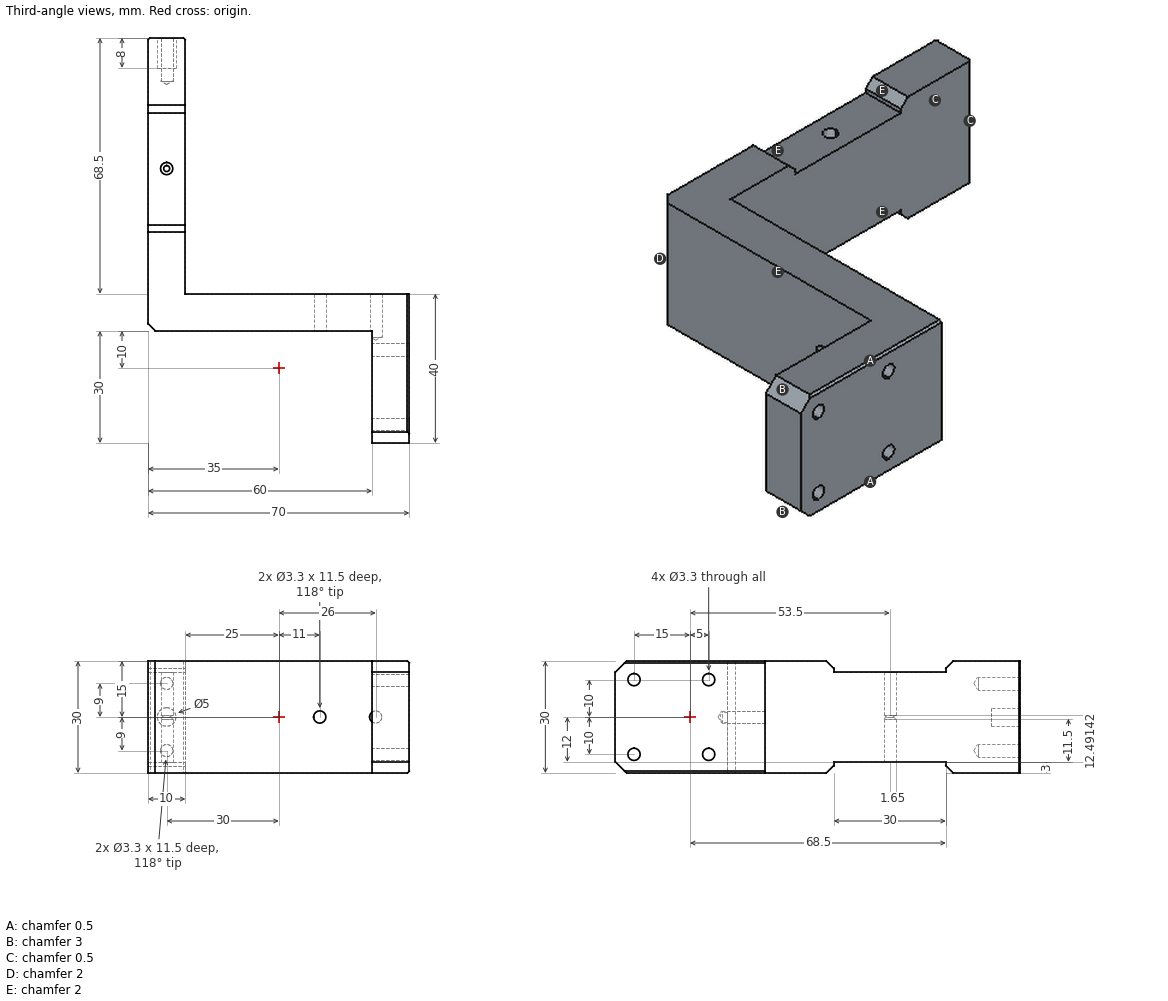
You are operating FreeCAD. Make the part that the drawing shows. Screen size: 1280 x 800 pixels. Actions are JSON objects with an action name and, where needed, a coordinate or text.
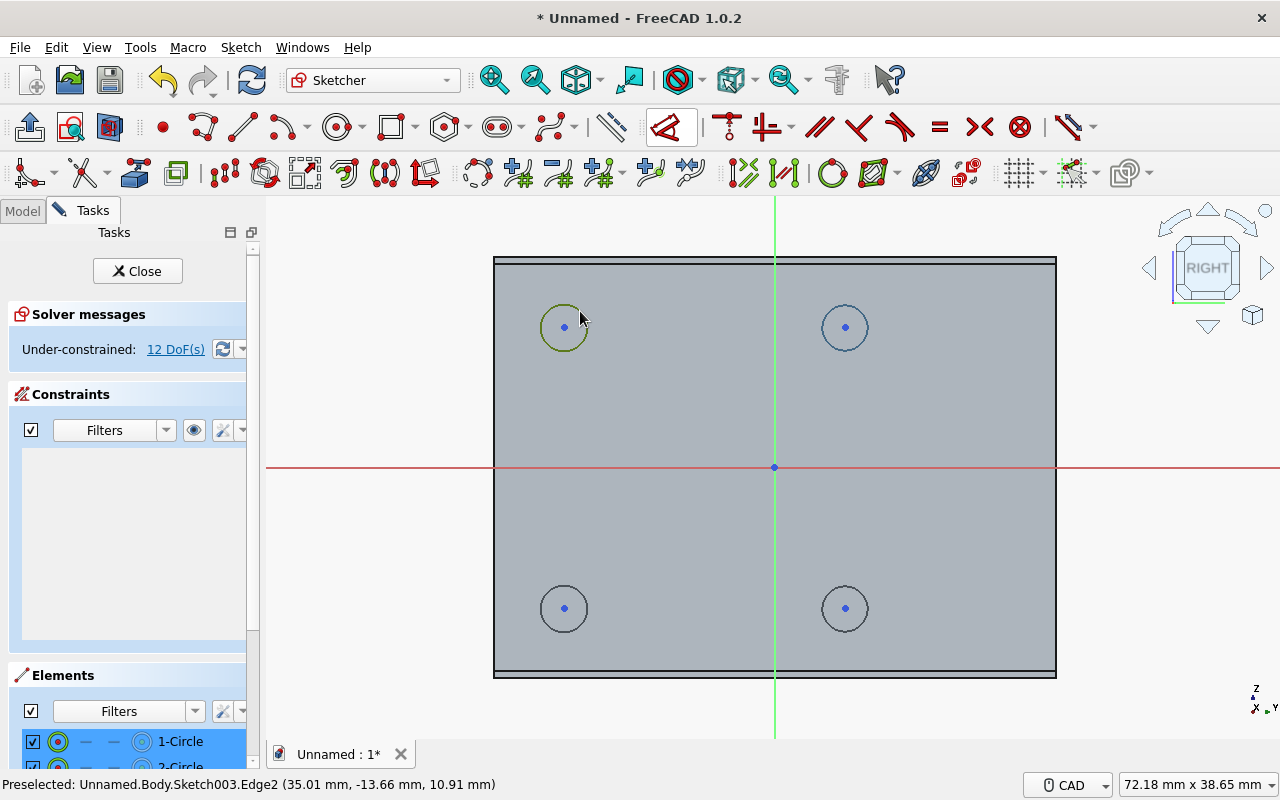
{"action": "left_click", "coordinate": [580, 592]}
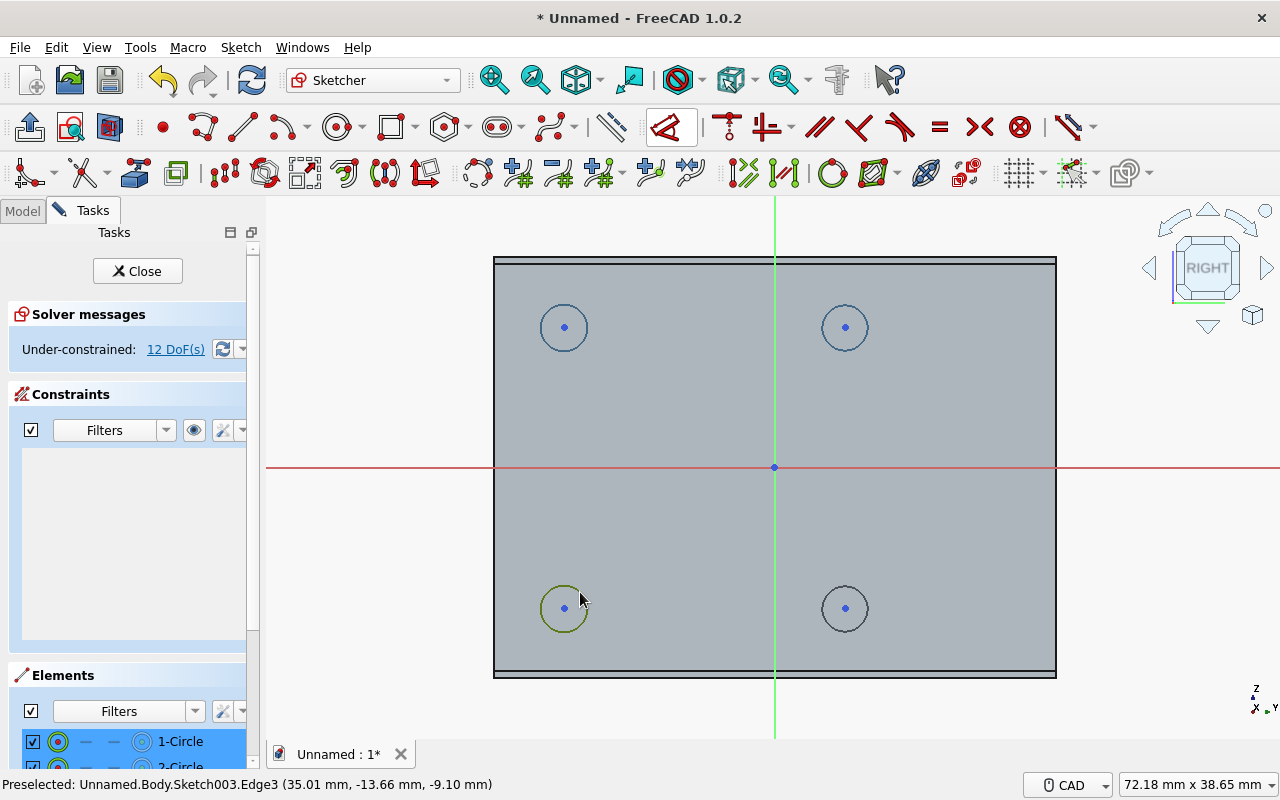
{"action": "left_click", "coordinate": [861, 593]}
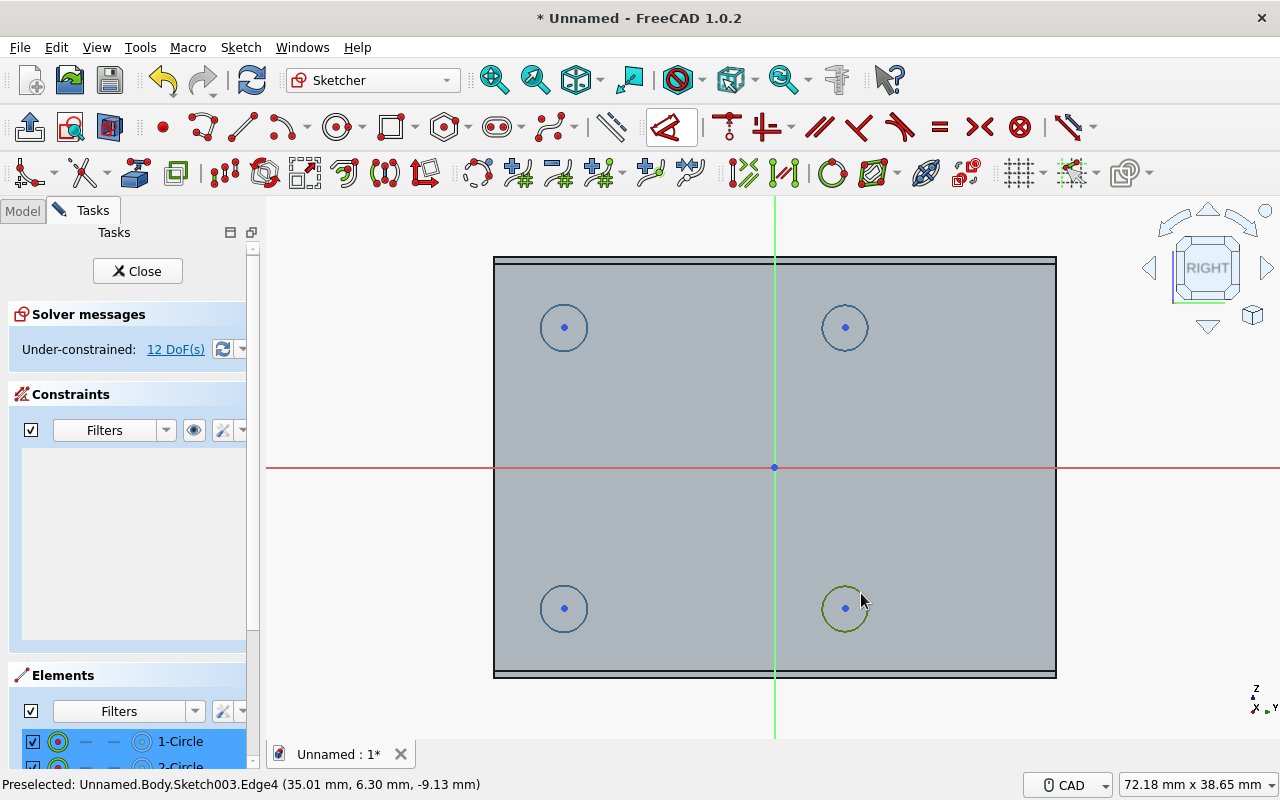
{"action": "key", "text": "e"}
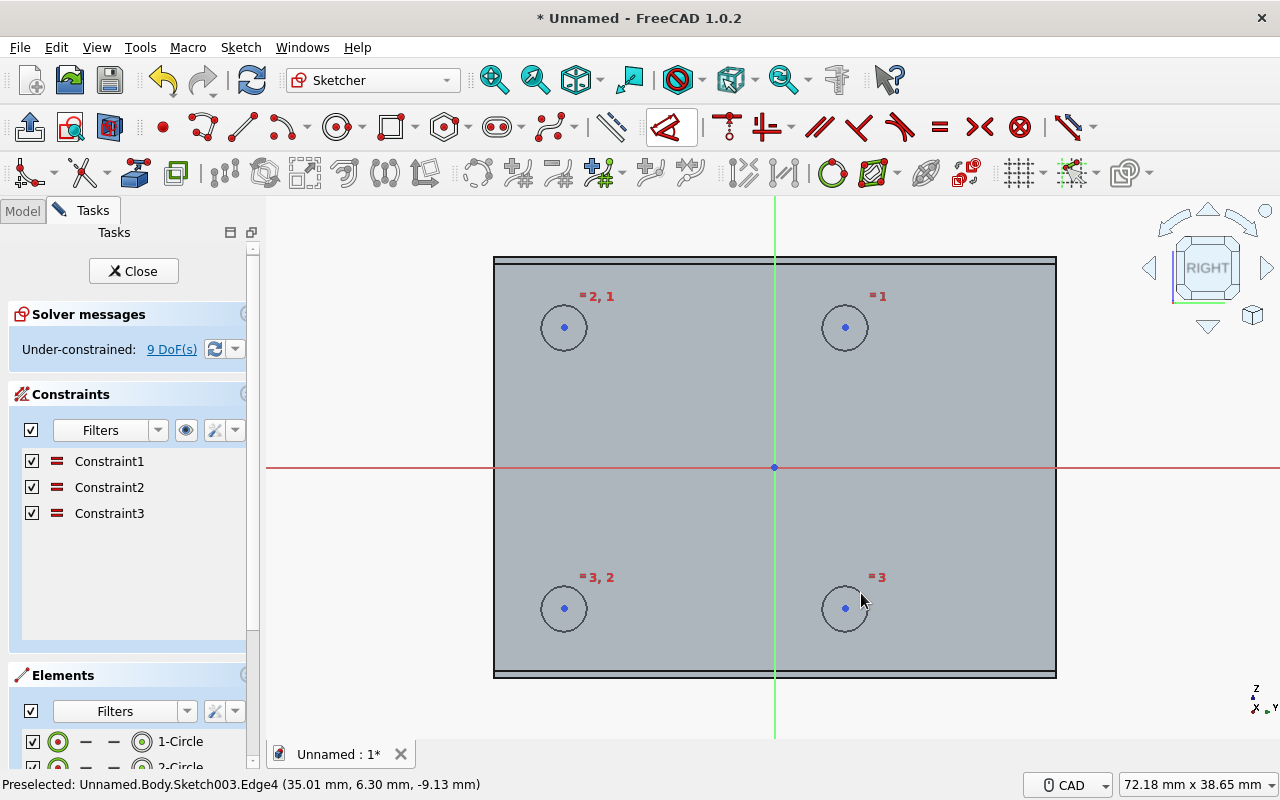
{"action": "left_click", "coordinate": [861, 312]}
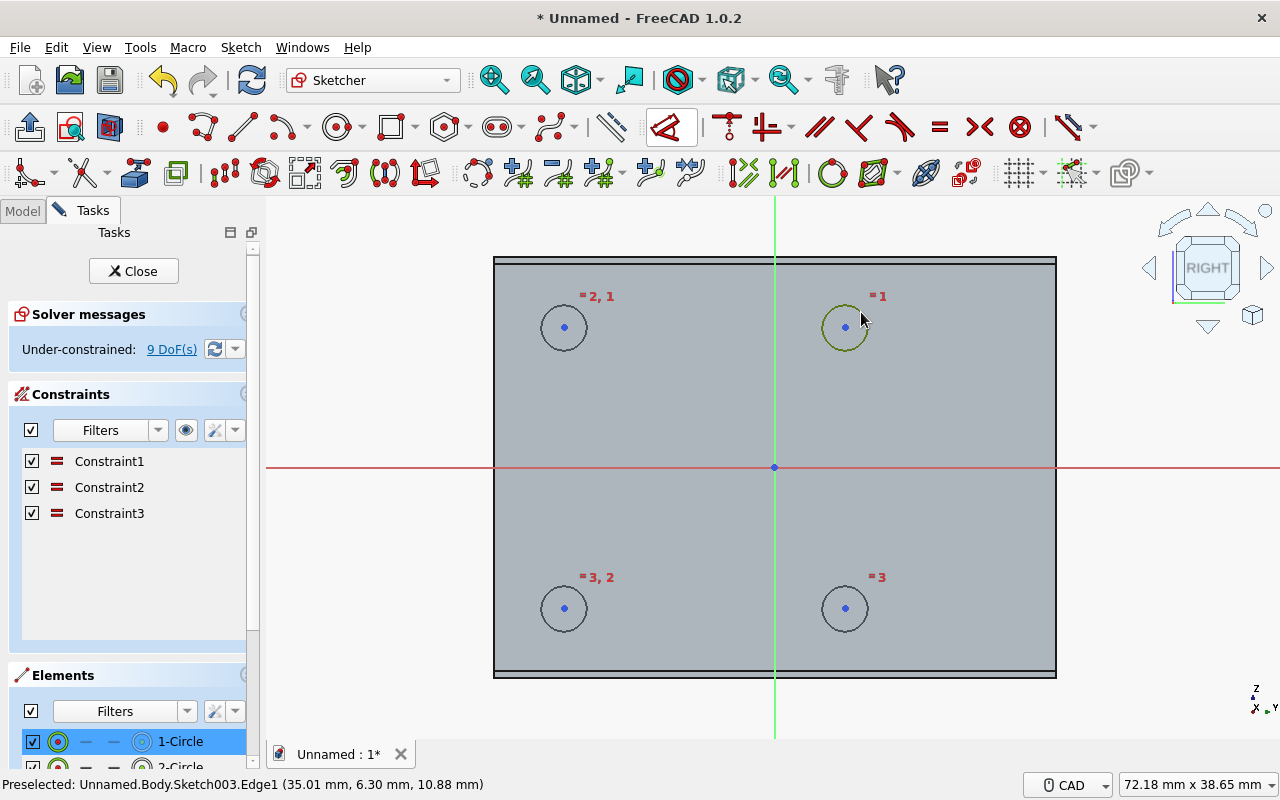
{"action": "left_click", "coordinate": [692, 128]}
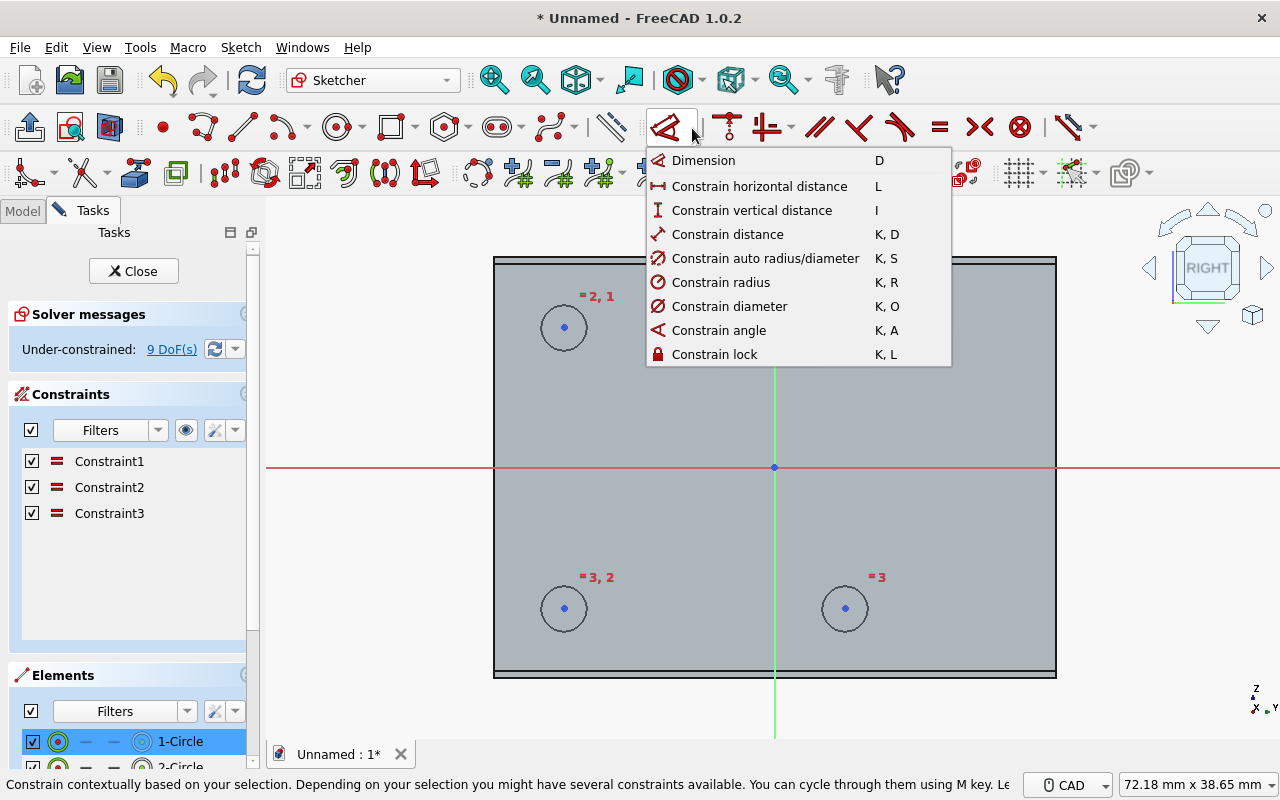
{"action": "left_click", "coordinate": [799, 306]}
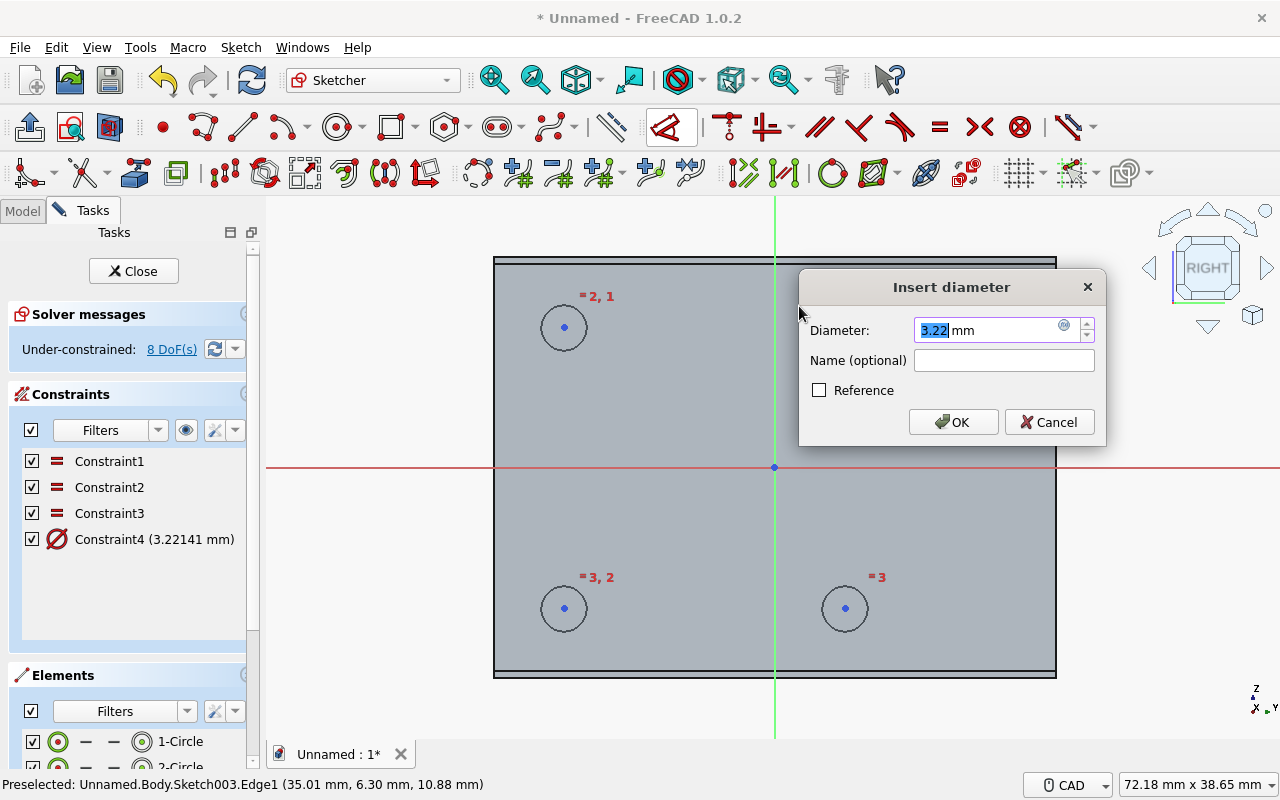
{"action": "type", "text": "3.3"}
{"action": "key", "text": "Return"}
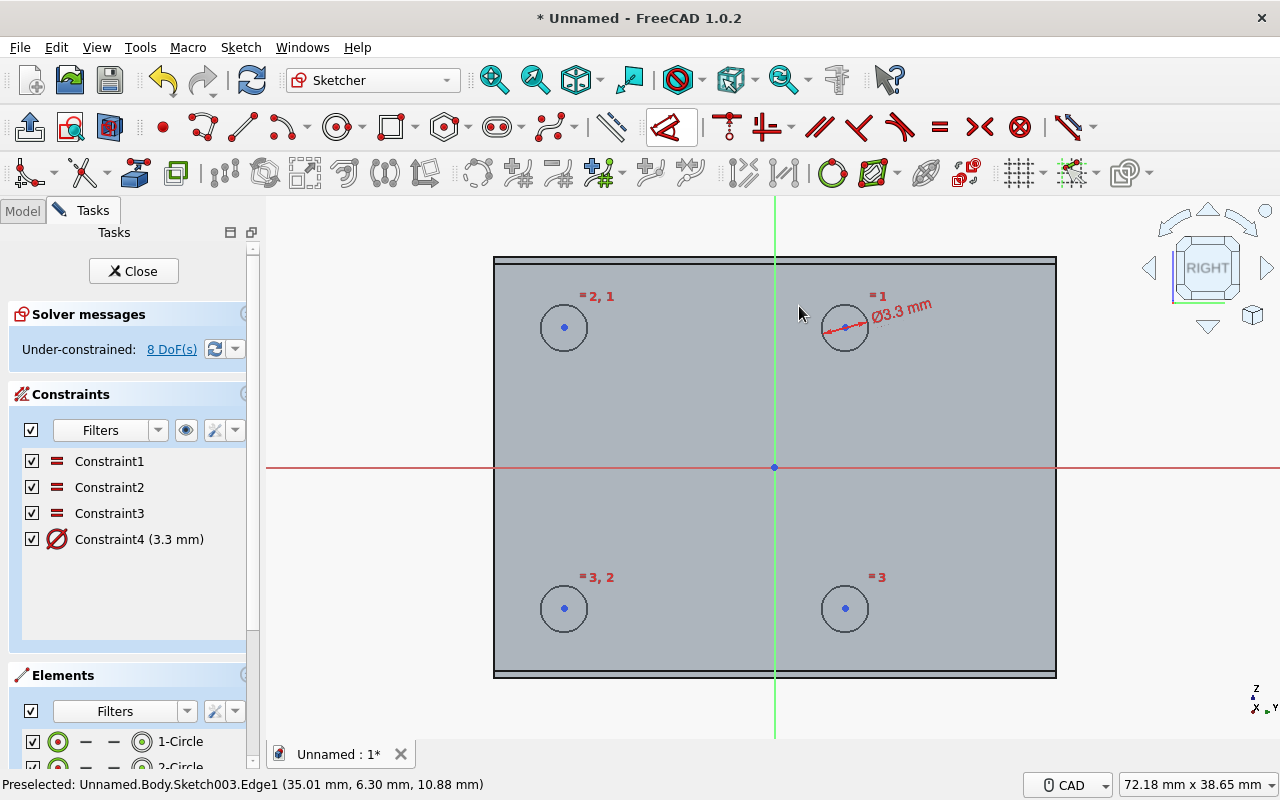
{"action": "left_click", "coordinate": [845, 328]}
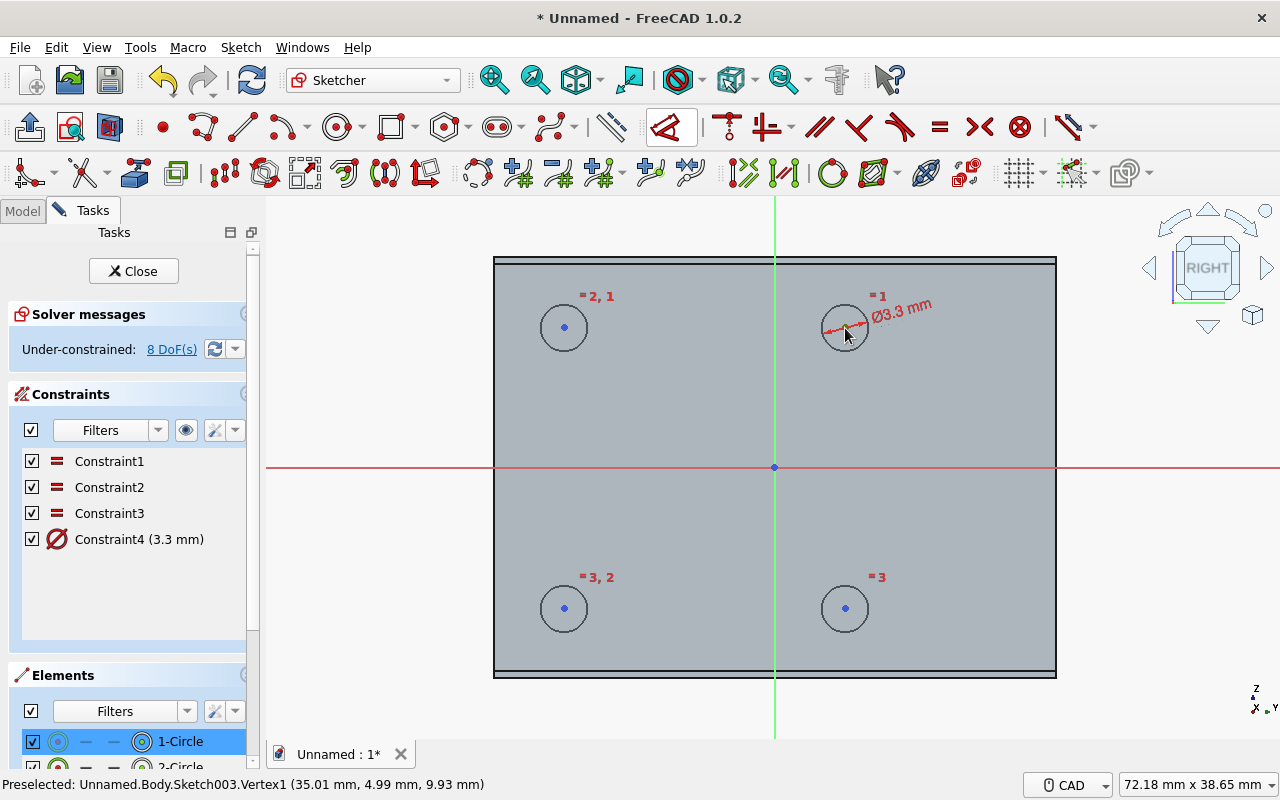
{"action": "left_click", "coordinate": [692, 128]}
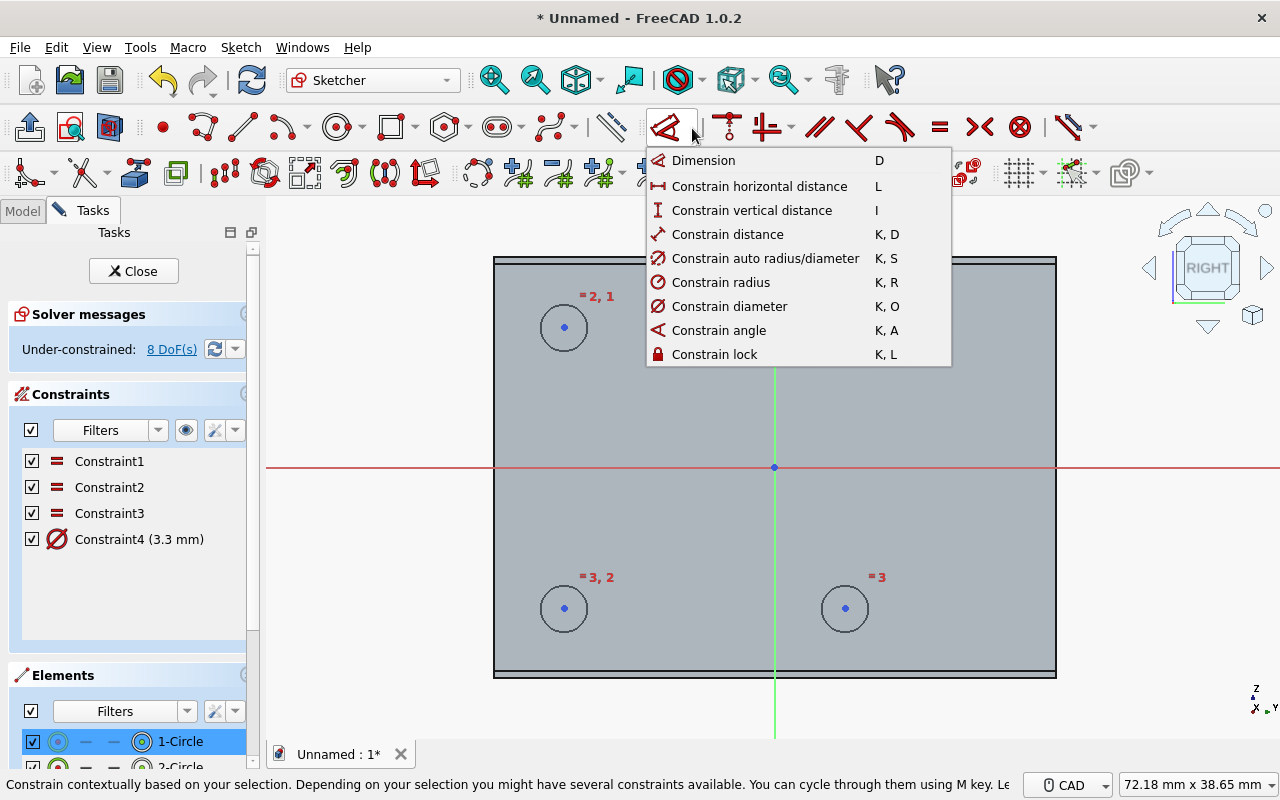
{"action": "left_click", "coordinate": [799, 186]}